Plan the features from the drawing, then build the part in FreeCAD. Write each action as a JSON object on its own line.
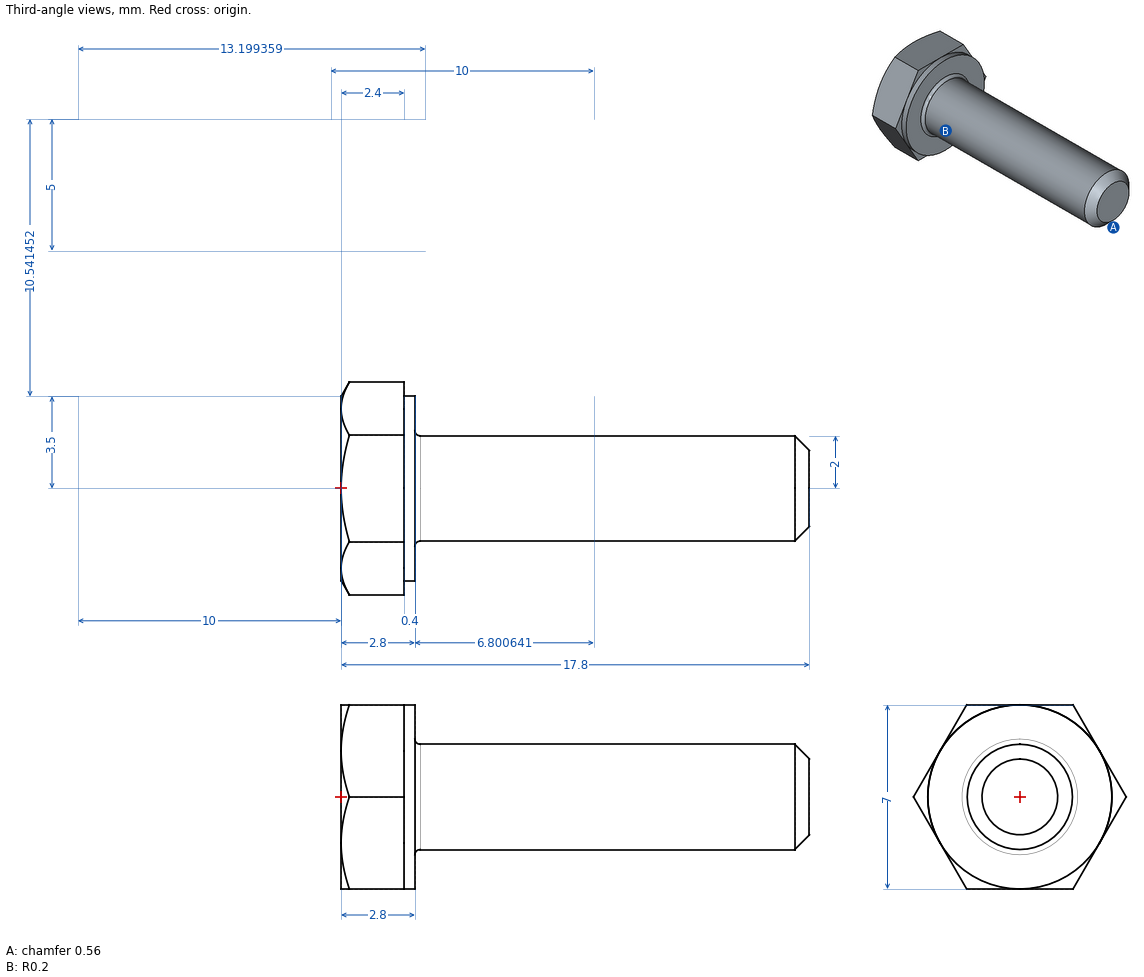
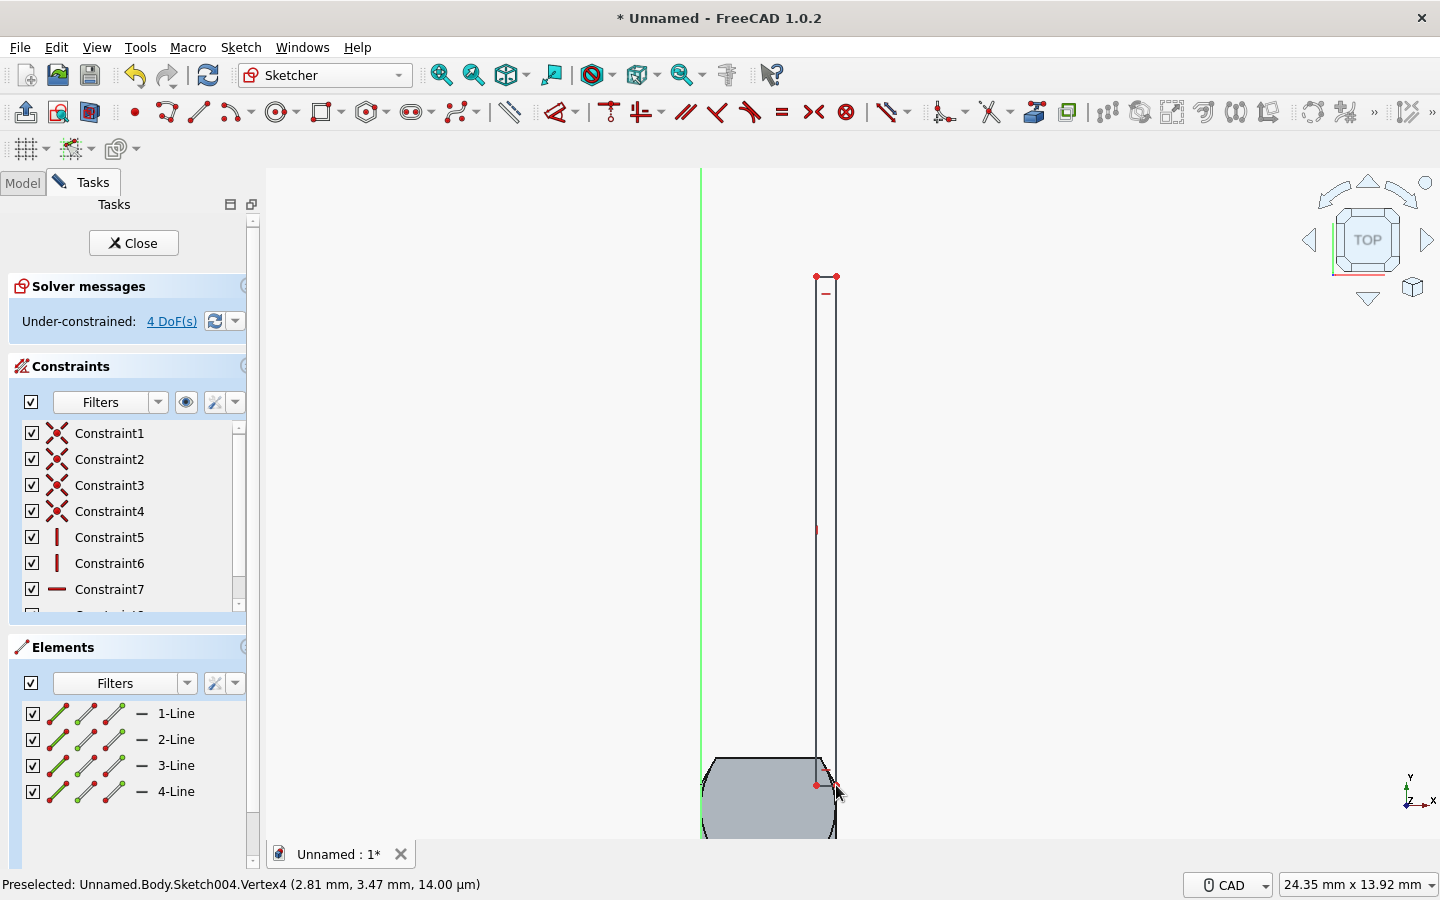
{"action": "key", "text": "d"}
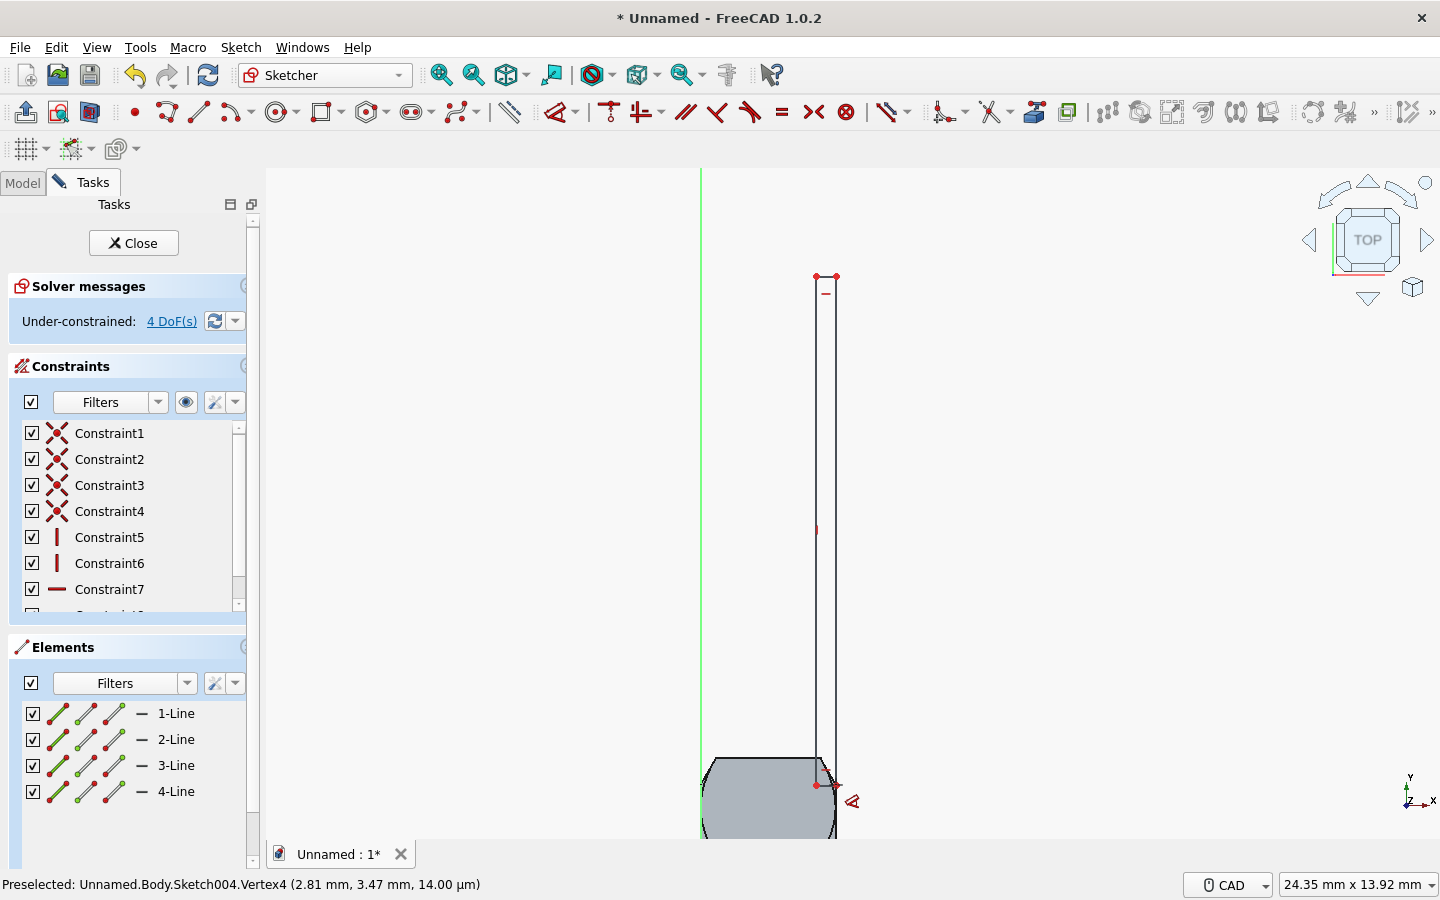
{"action": "scroll", "coordinate": [826, 786], "scroll_direction": "up", "scroll_amount": 4}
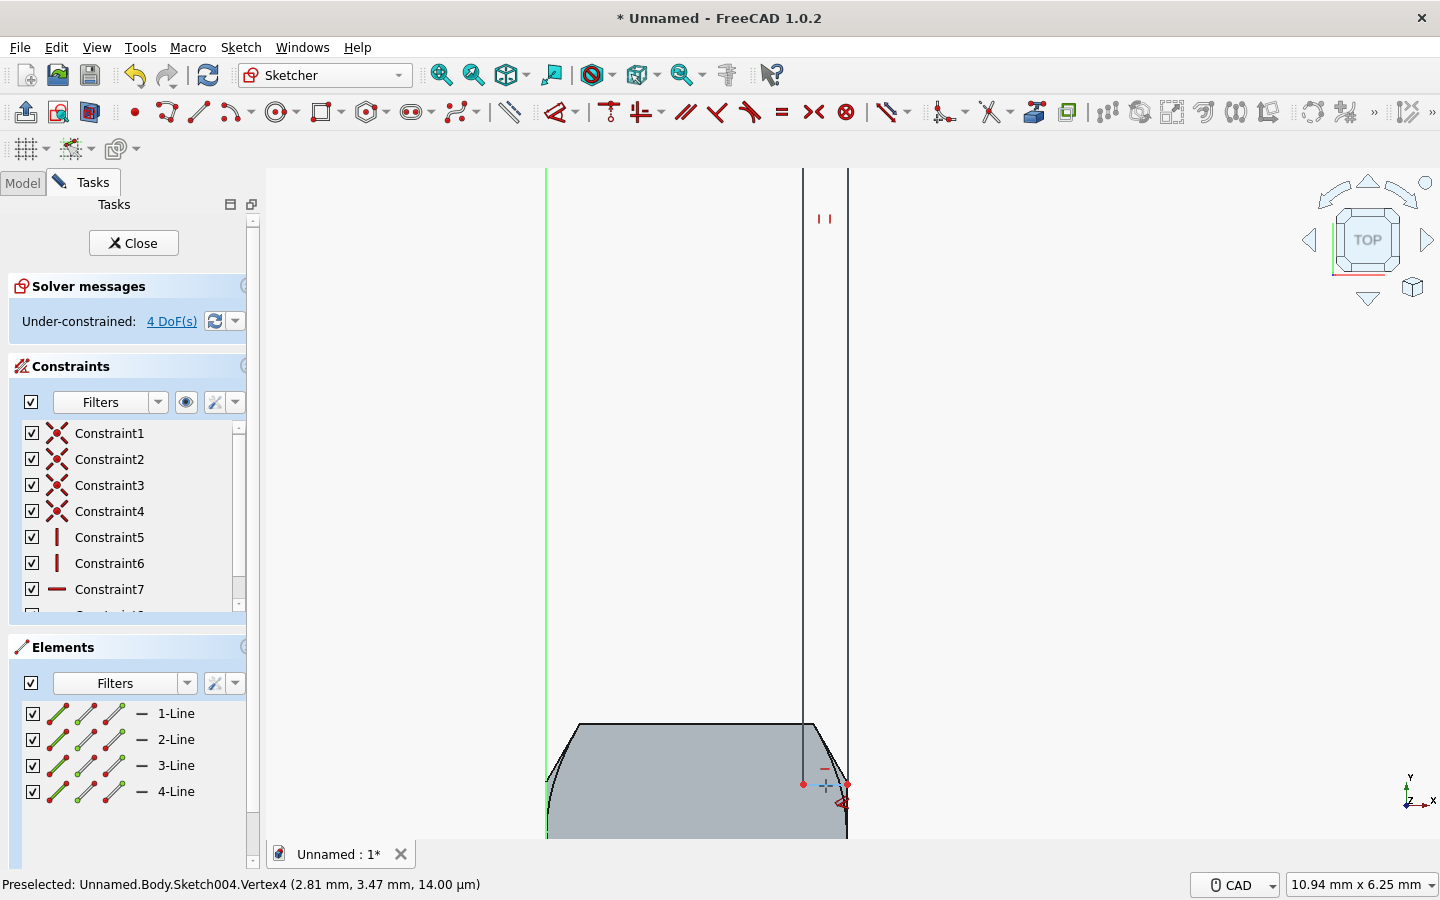
{"action": "left_click", "coordinate": [825, 785]}
{"action": "left_click", "coordinate": [825, 751]}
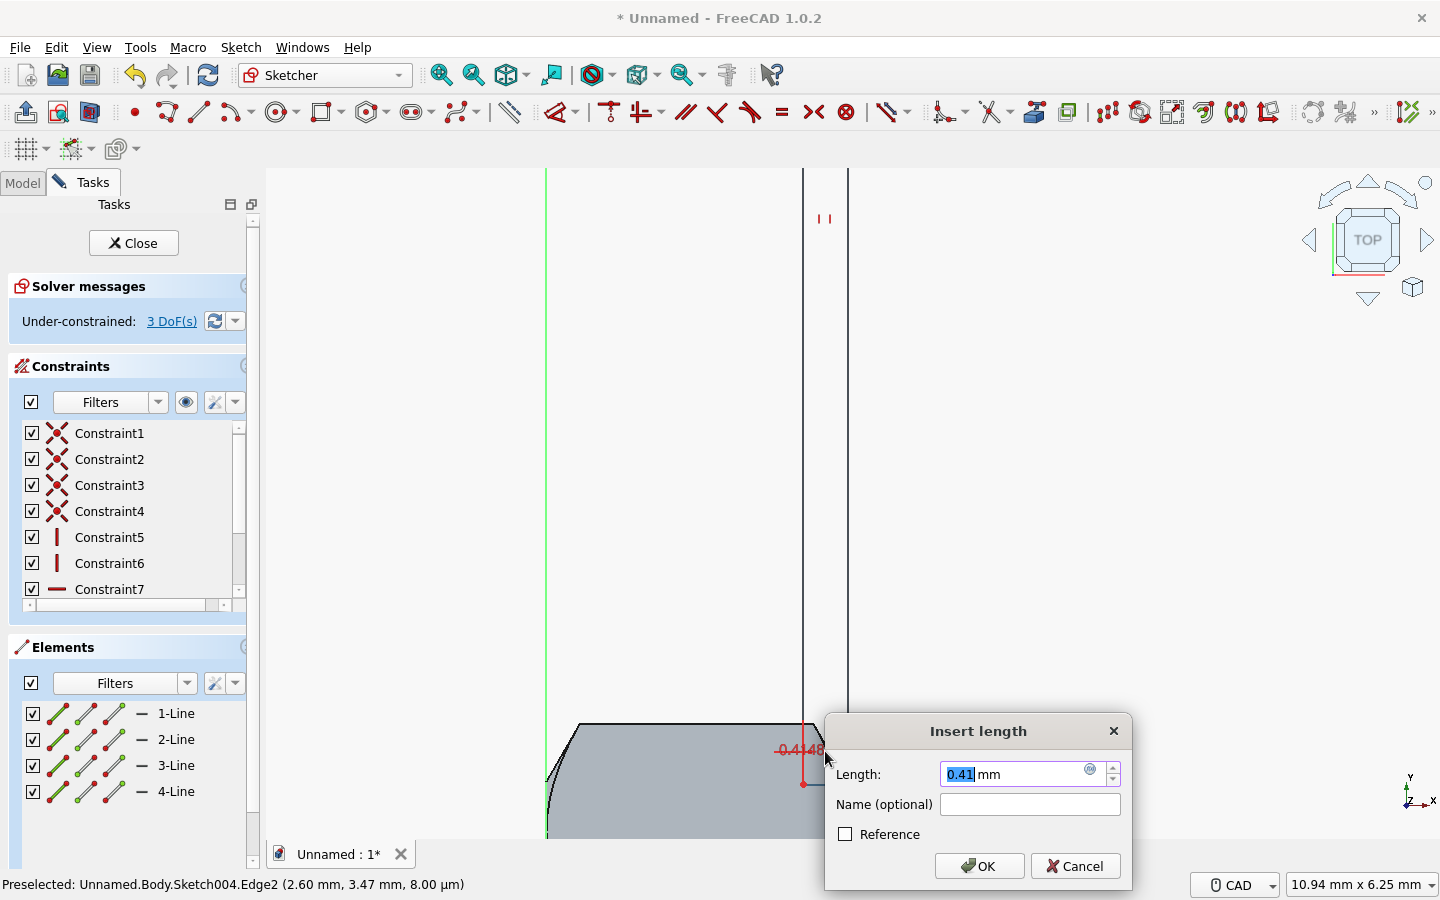
{"action": "type", "text": "0.4"}
{"action": "key", "text": "Return"}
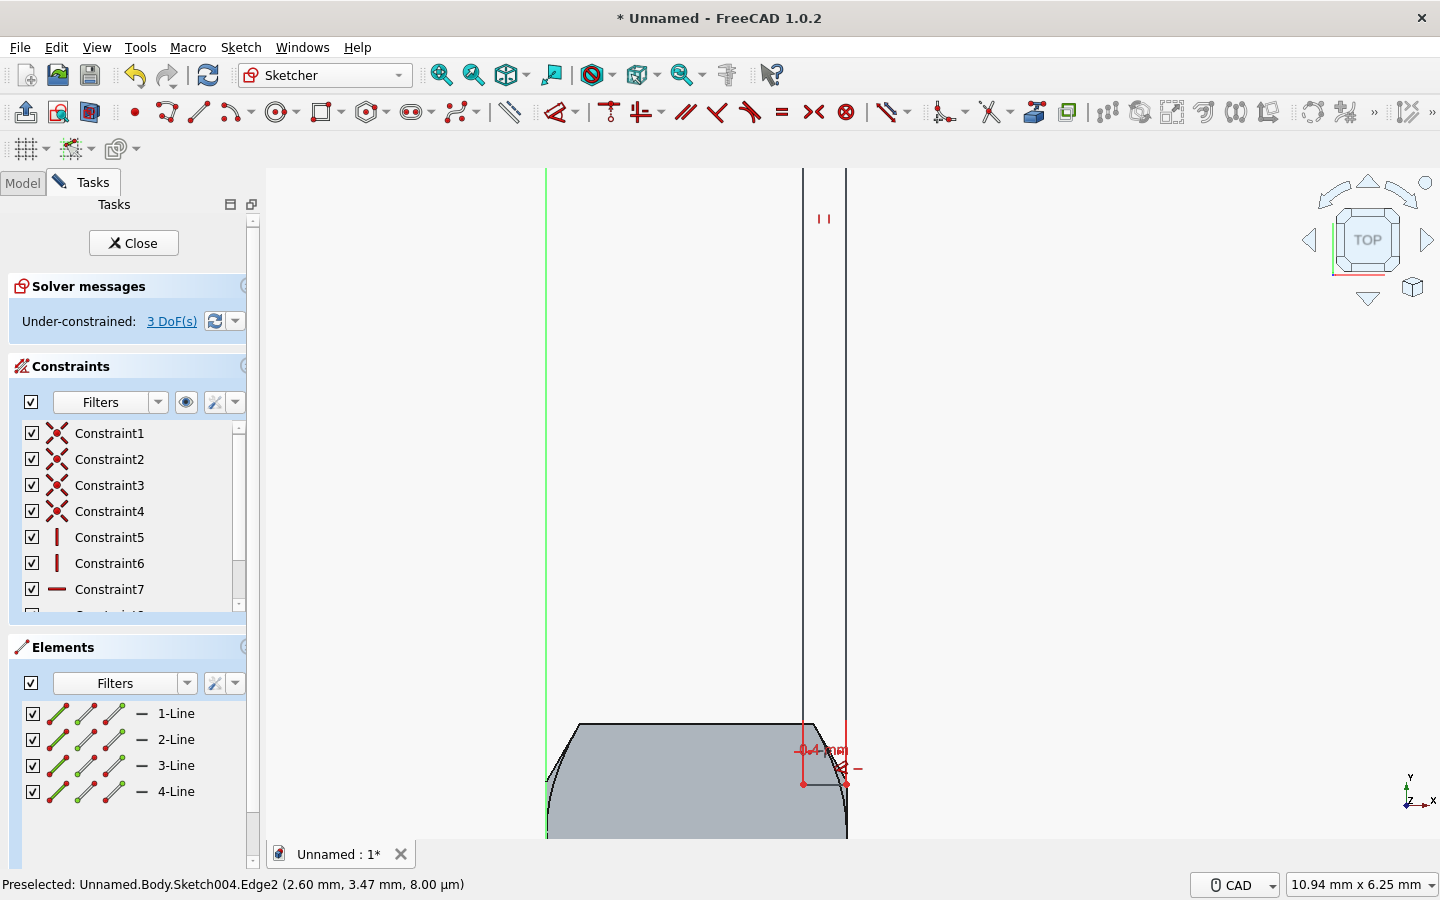
{"action": "scroll", "coordinate": [822, 546], "scroll_direction": "down", "scroll_amount": 6}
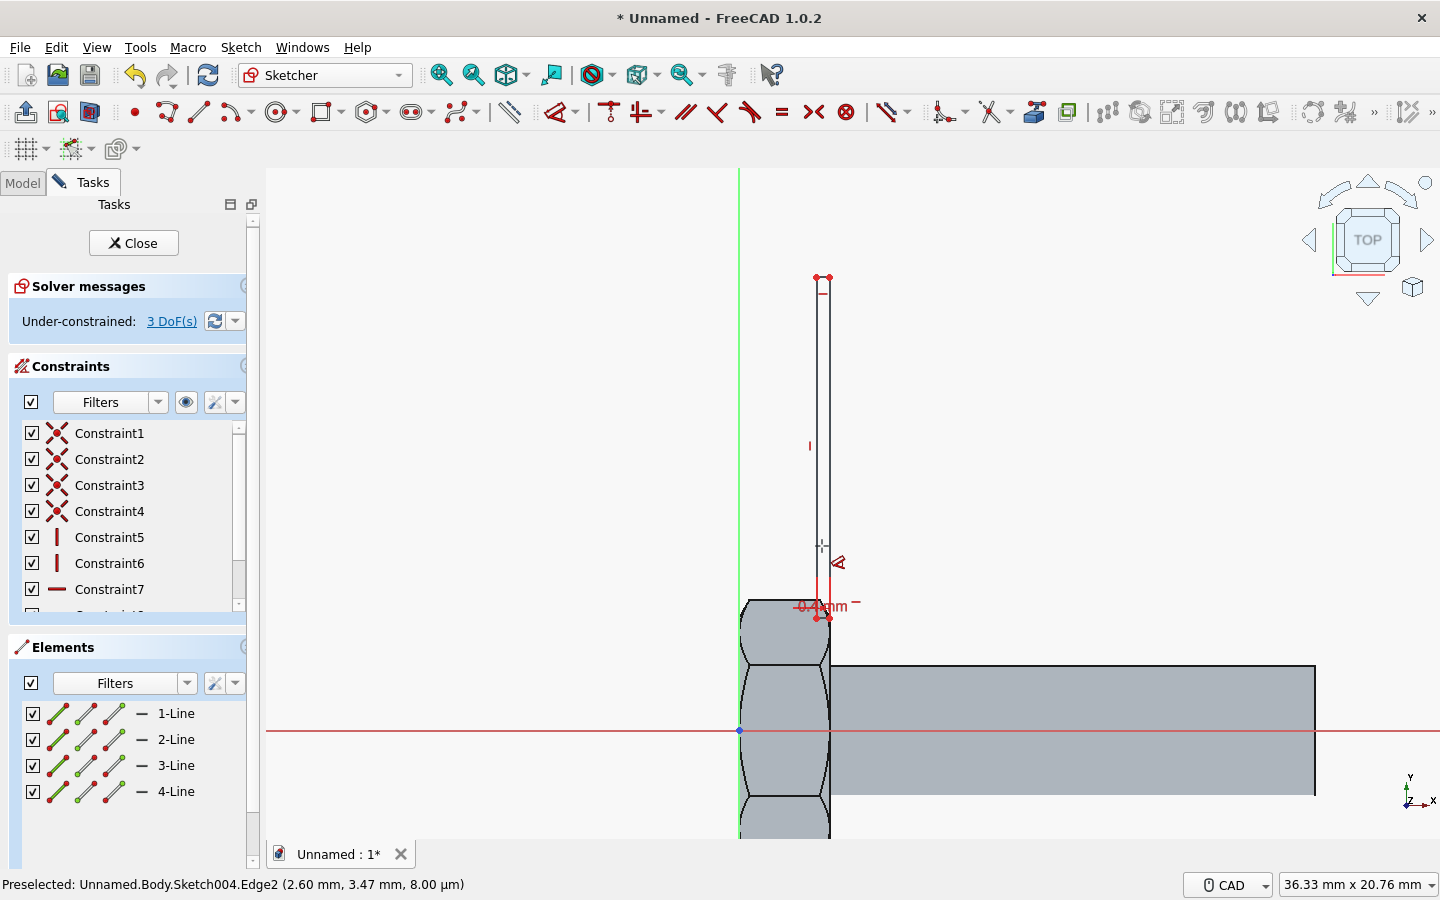
{"action": "left_click", "coordinate": [817, 277]}
{"action": "left_click", "coordinate": [778, 765]}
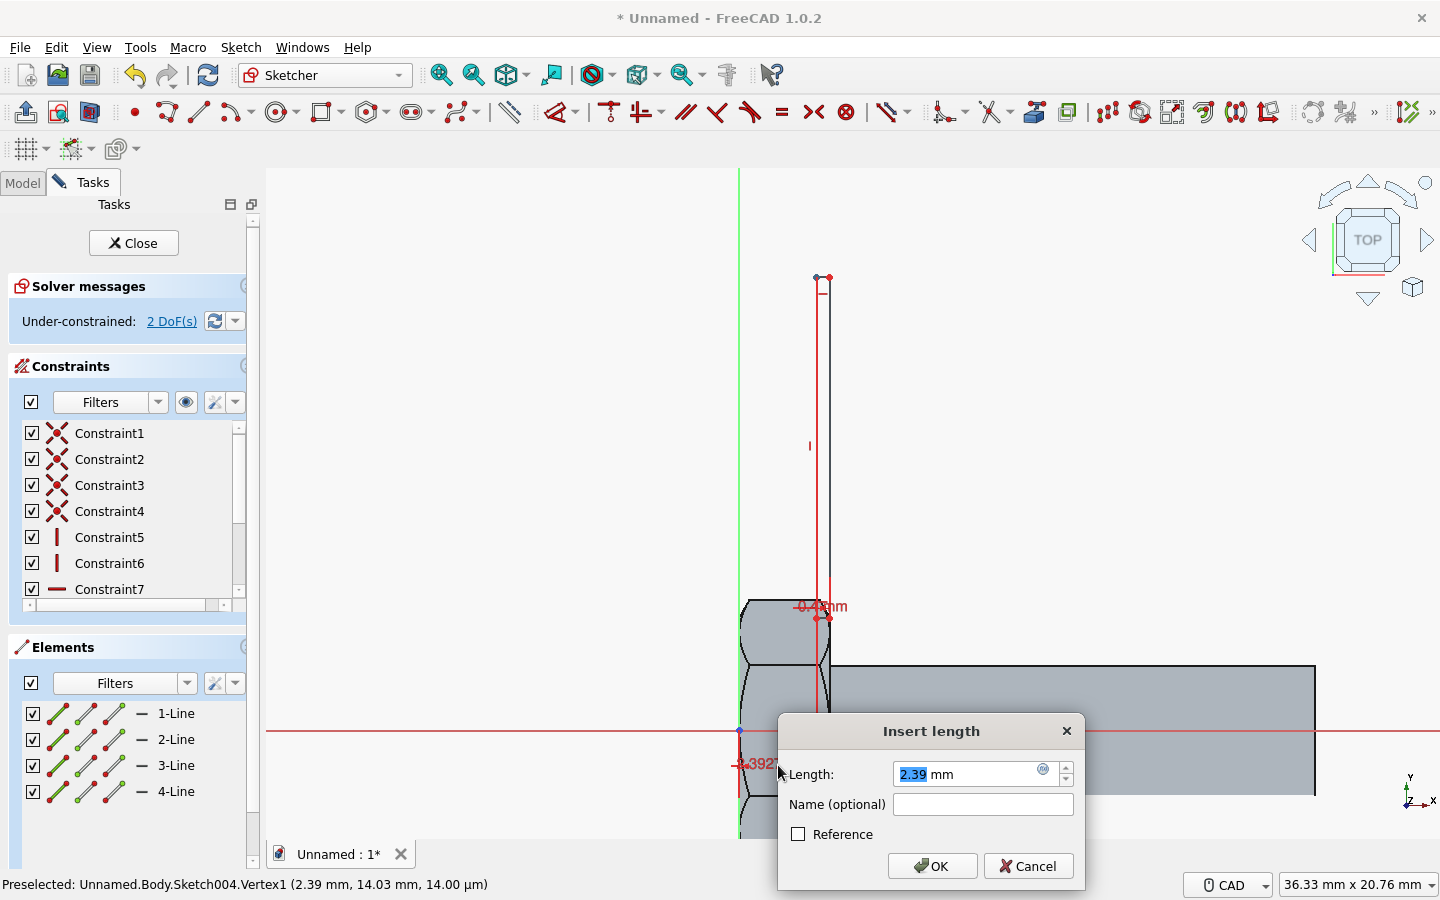
{"action": "type", "text": "2.4"}
{"action": "key", "text": "Return"}